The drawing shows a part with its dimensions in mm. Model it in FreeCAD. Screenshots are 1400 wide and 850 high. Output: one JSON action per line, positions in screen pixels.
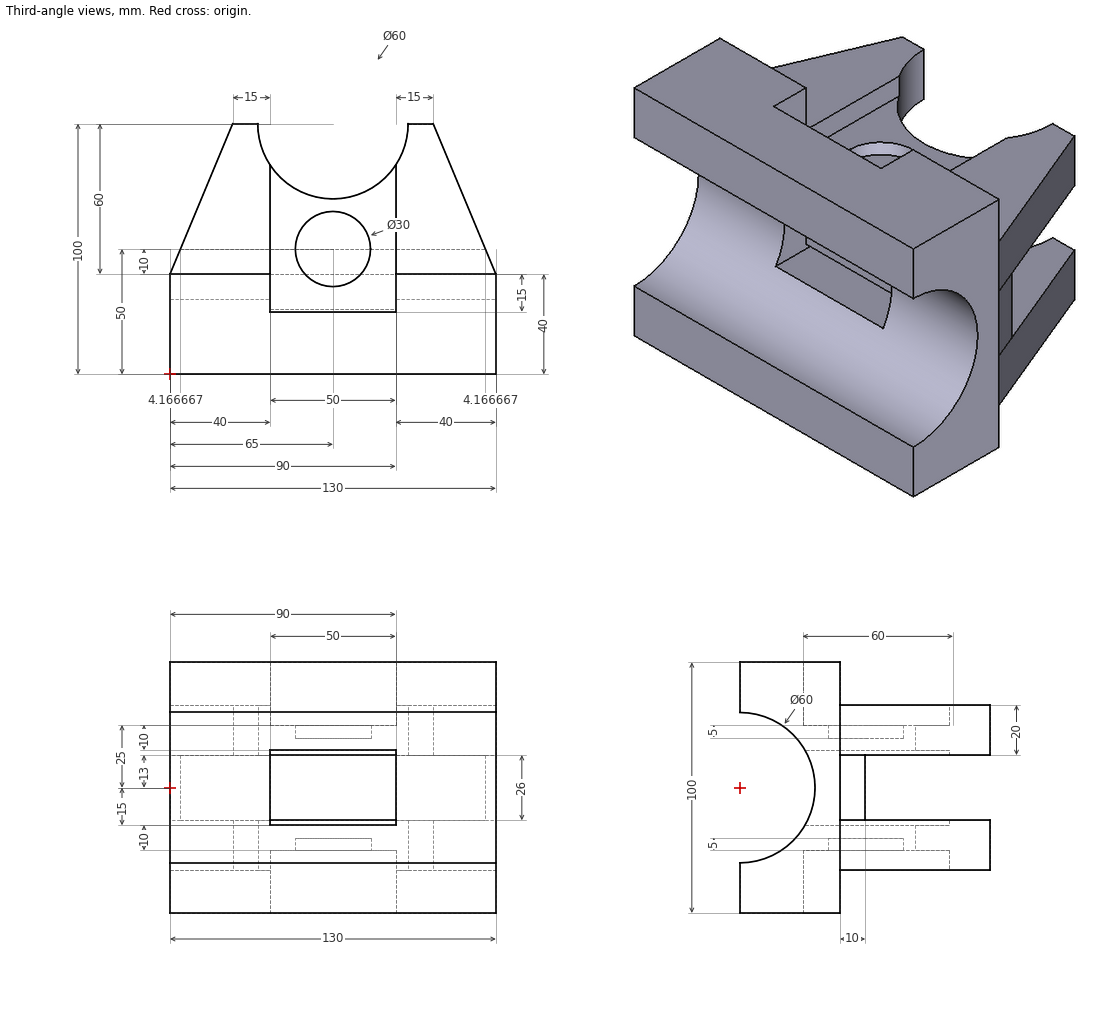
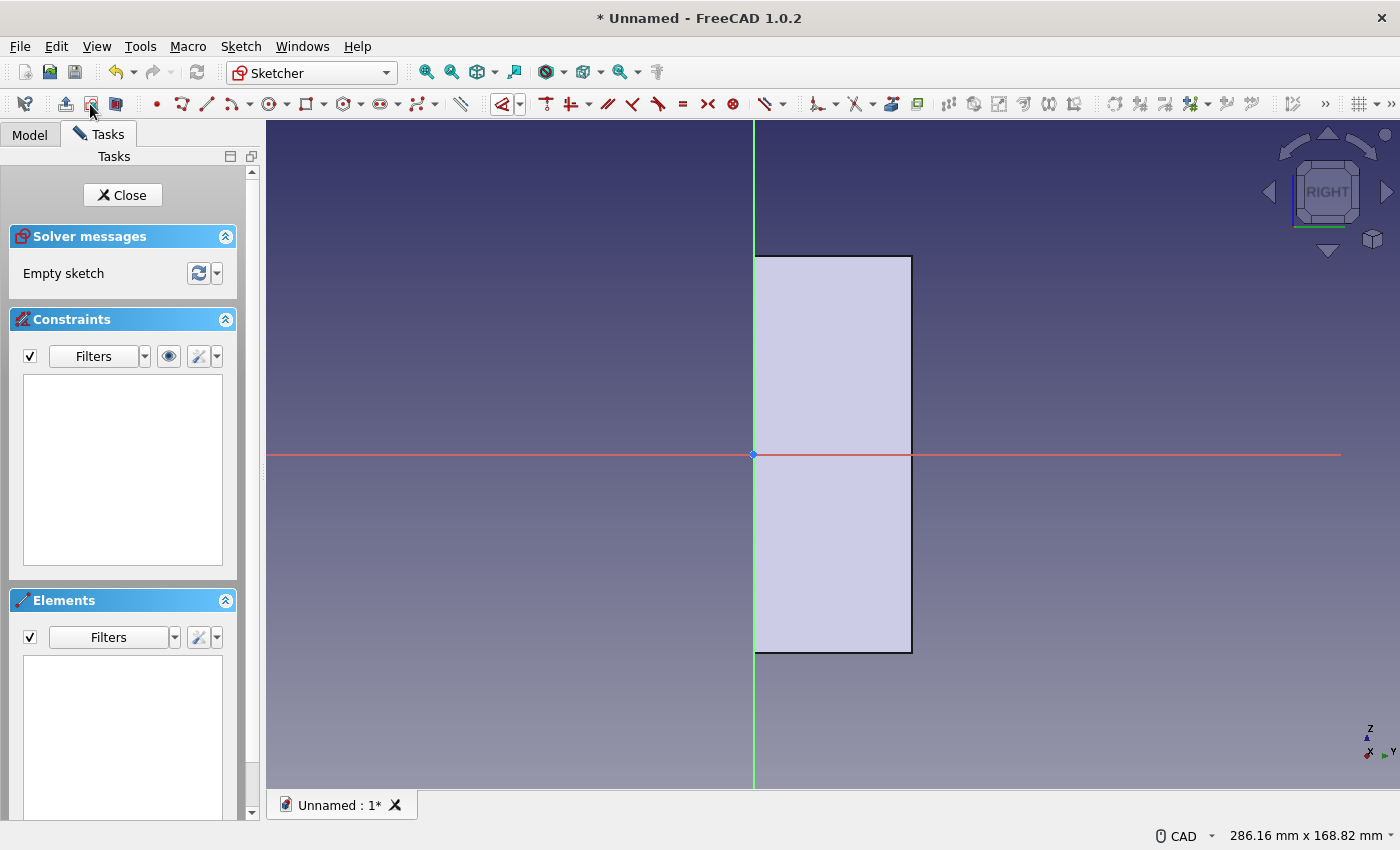
{"action": "scroll", "coordinate": [741, 454], "scroll_direction": "up", "scroll_amount": 3}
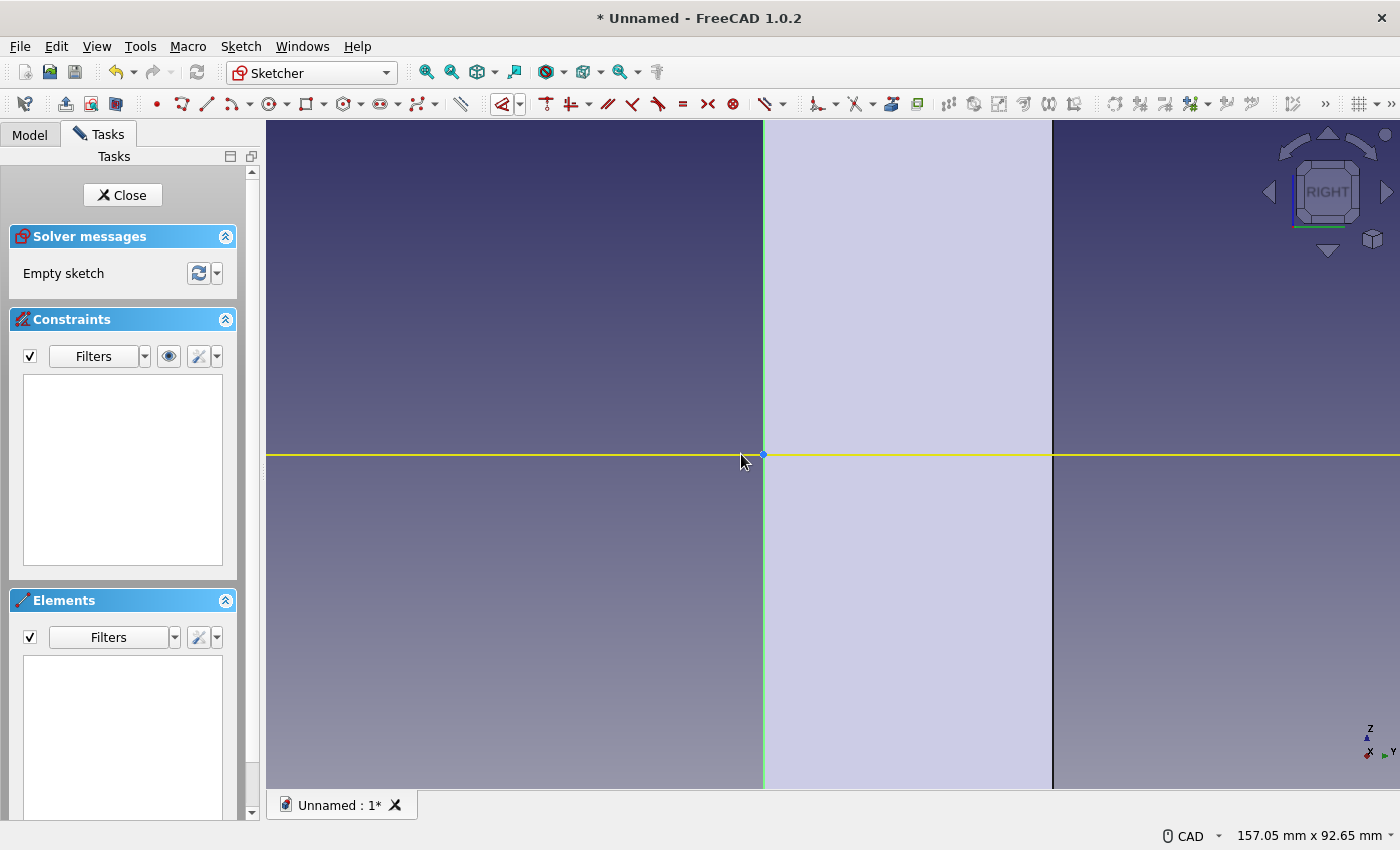
{"action": "left_click", "coordinate": [268, 104]}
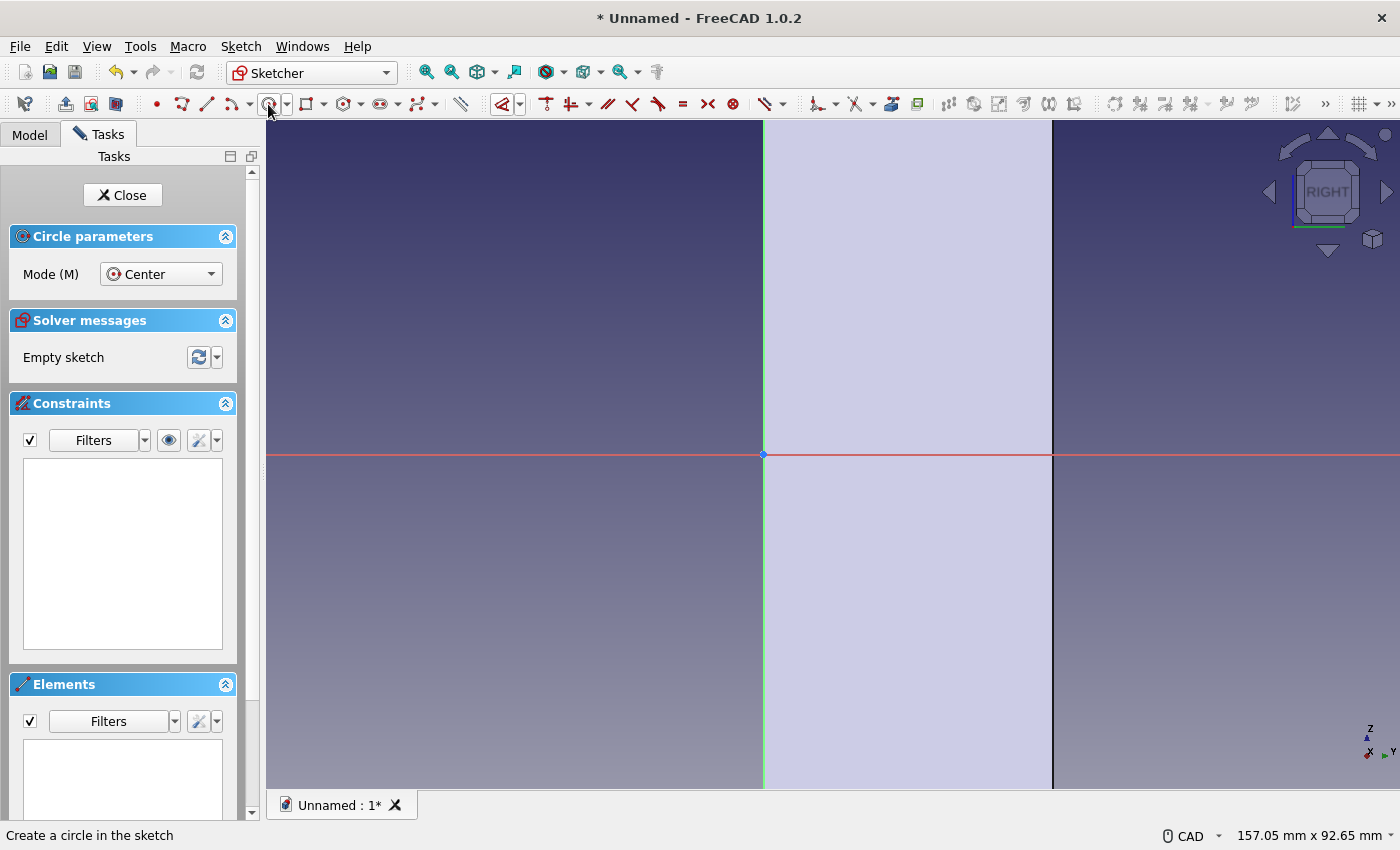
{"action": "left_click", "coordinate": [764, 454]}
{"action": "mouse_move", "coordinate": [917, 301]}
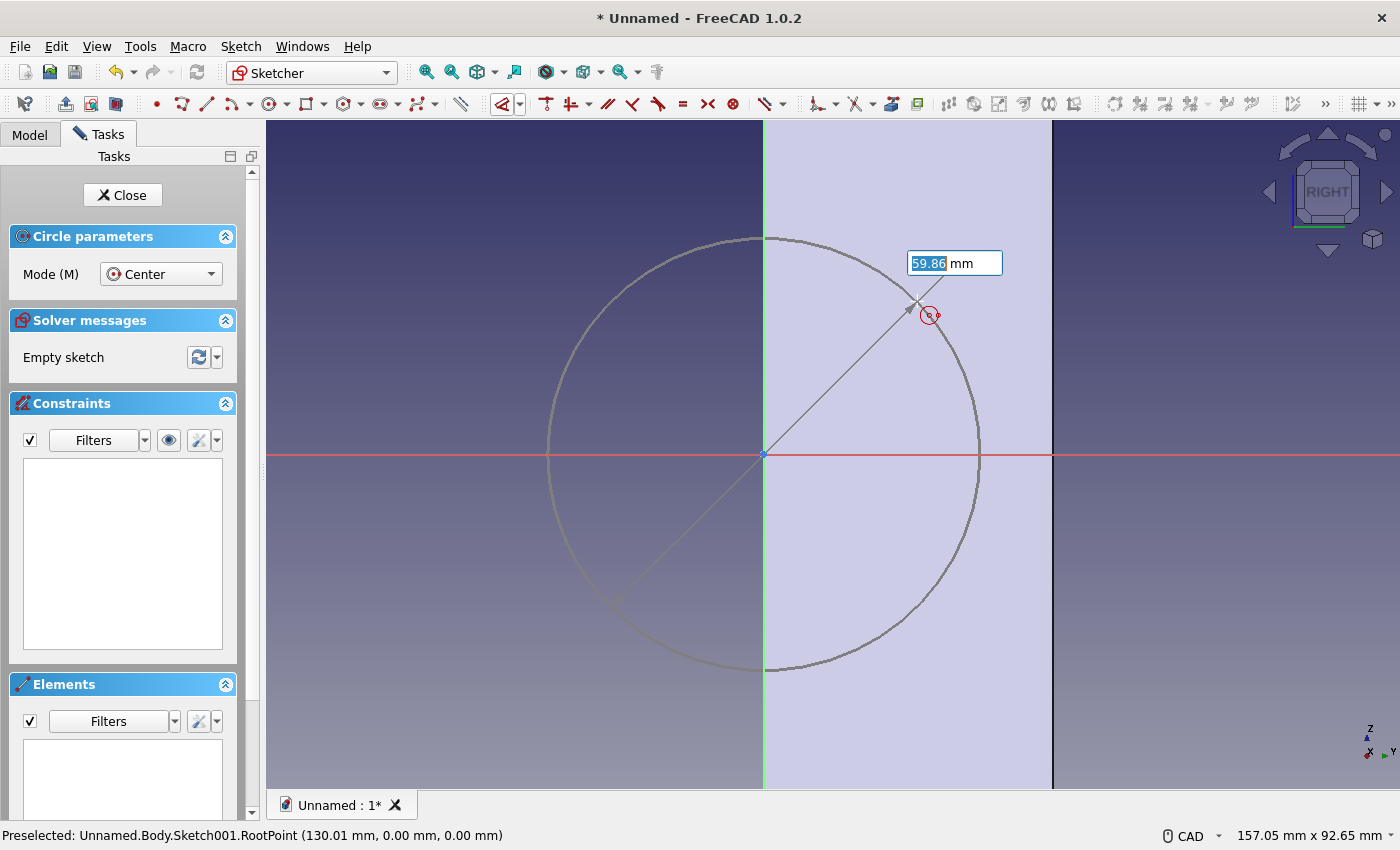
{"action": "type", "text": "60"}
{"action": "key", "text": "Return"}
{"action": "key", "text": "Escape"}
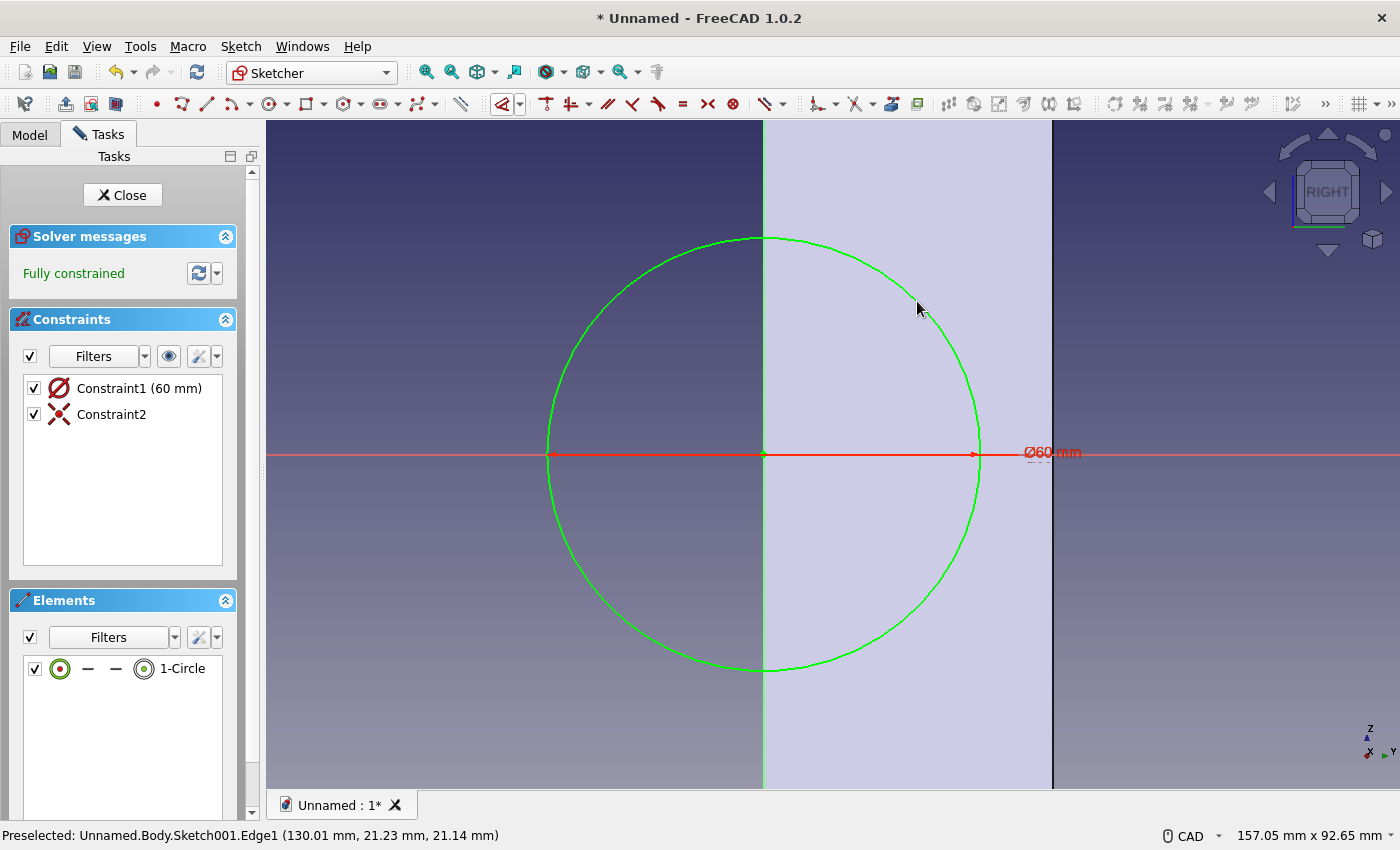
{"action": "left_click", "coordinate": [123, 195]}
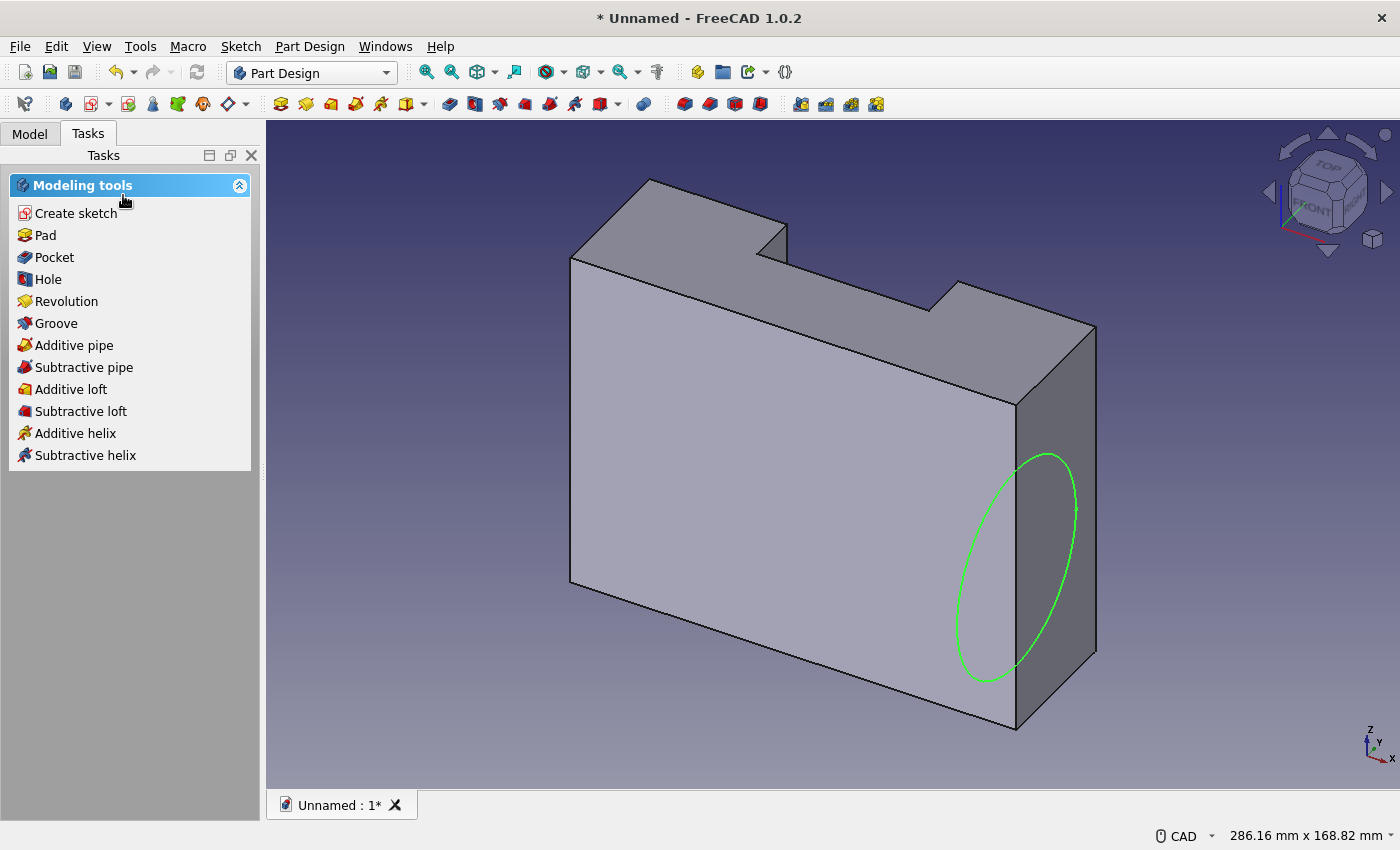
{"action": "left_click", "coordinate": [450, 104]}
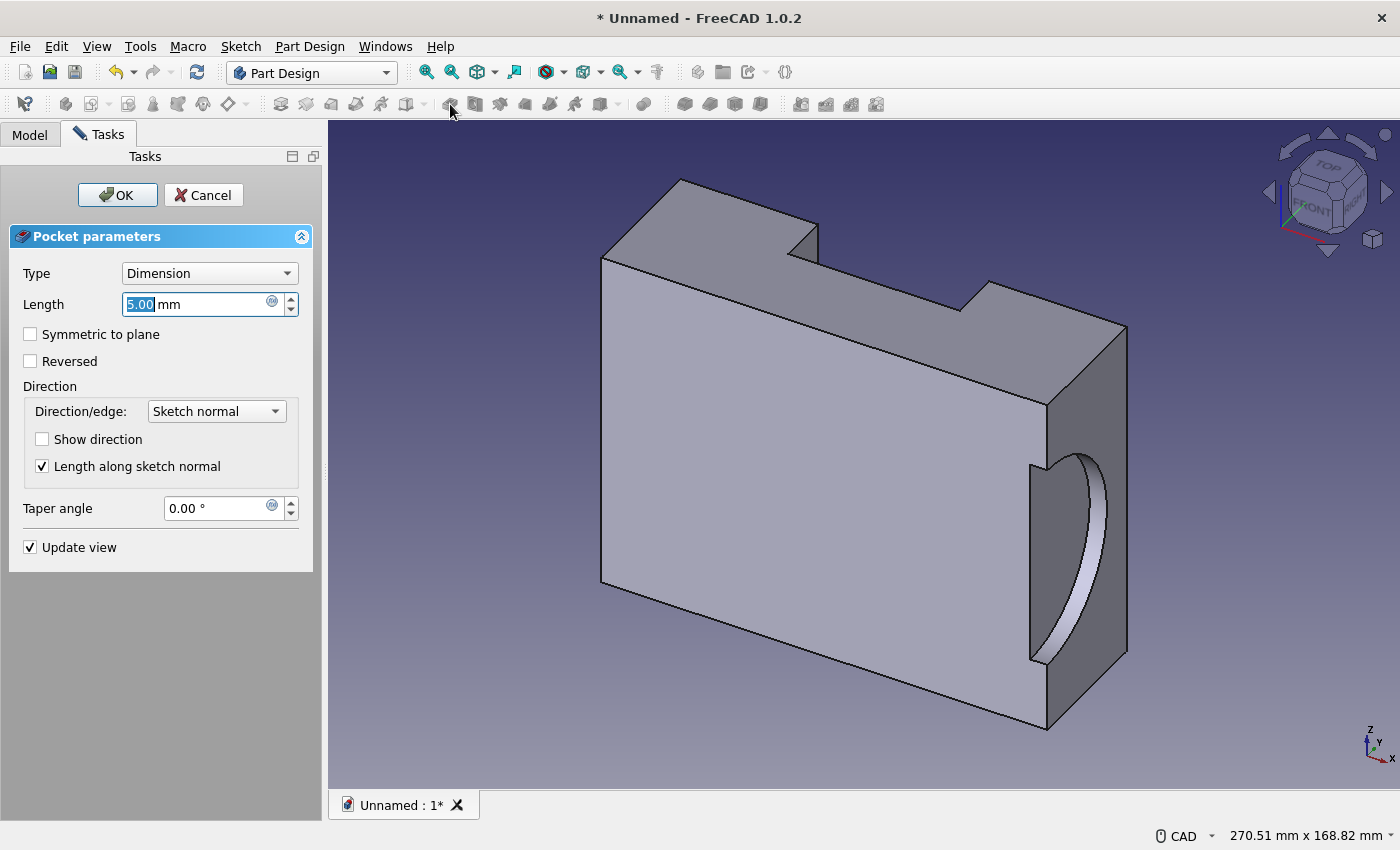
{"action": "left_click", "coordinate": [210, 274]}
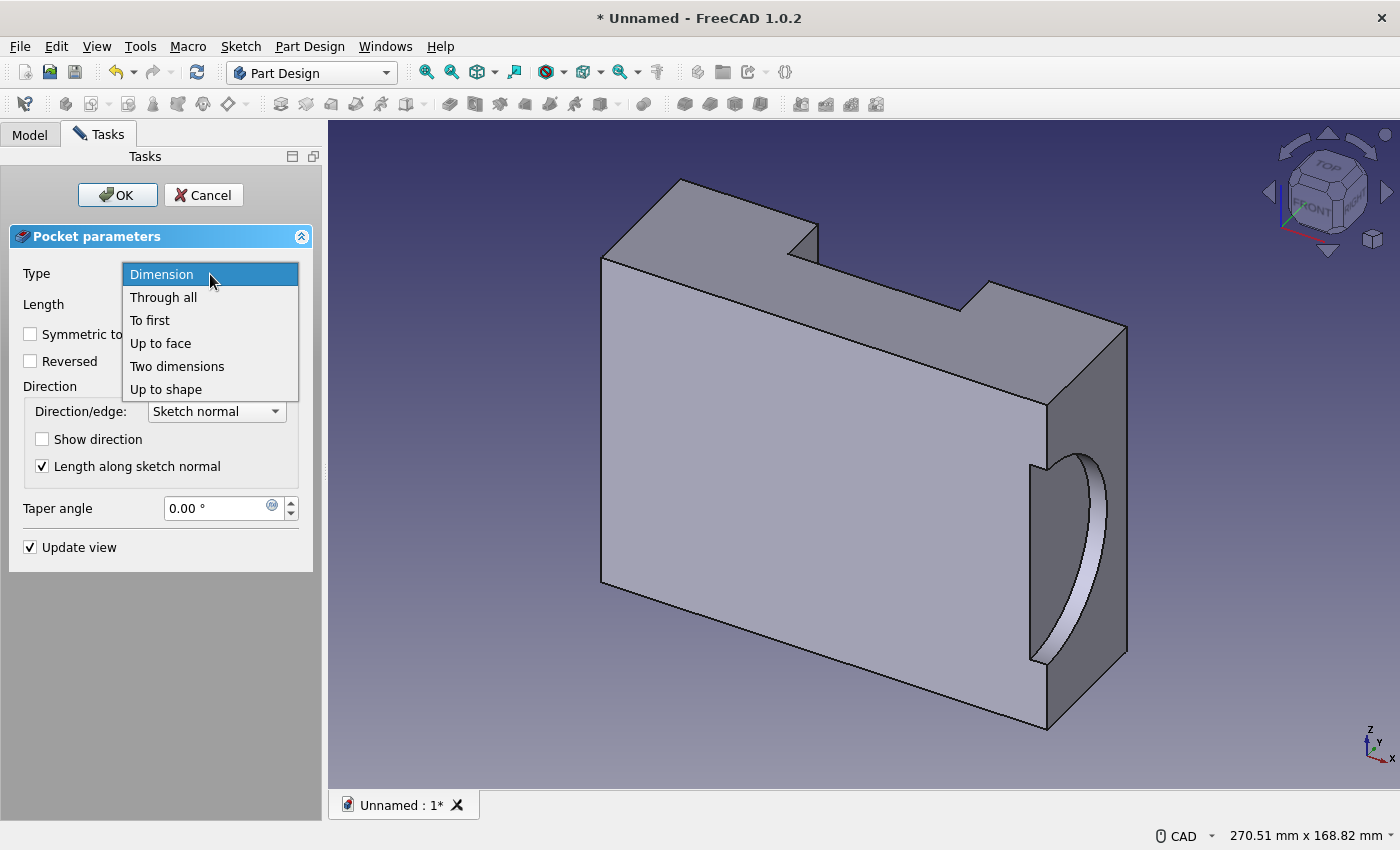
{"action": "left_click", "coordinate": [208, 298]}